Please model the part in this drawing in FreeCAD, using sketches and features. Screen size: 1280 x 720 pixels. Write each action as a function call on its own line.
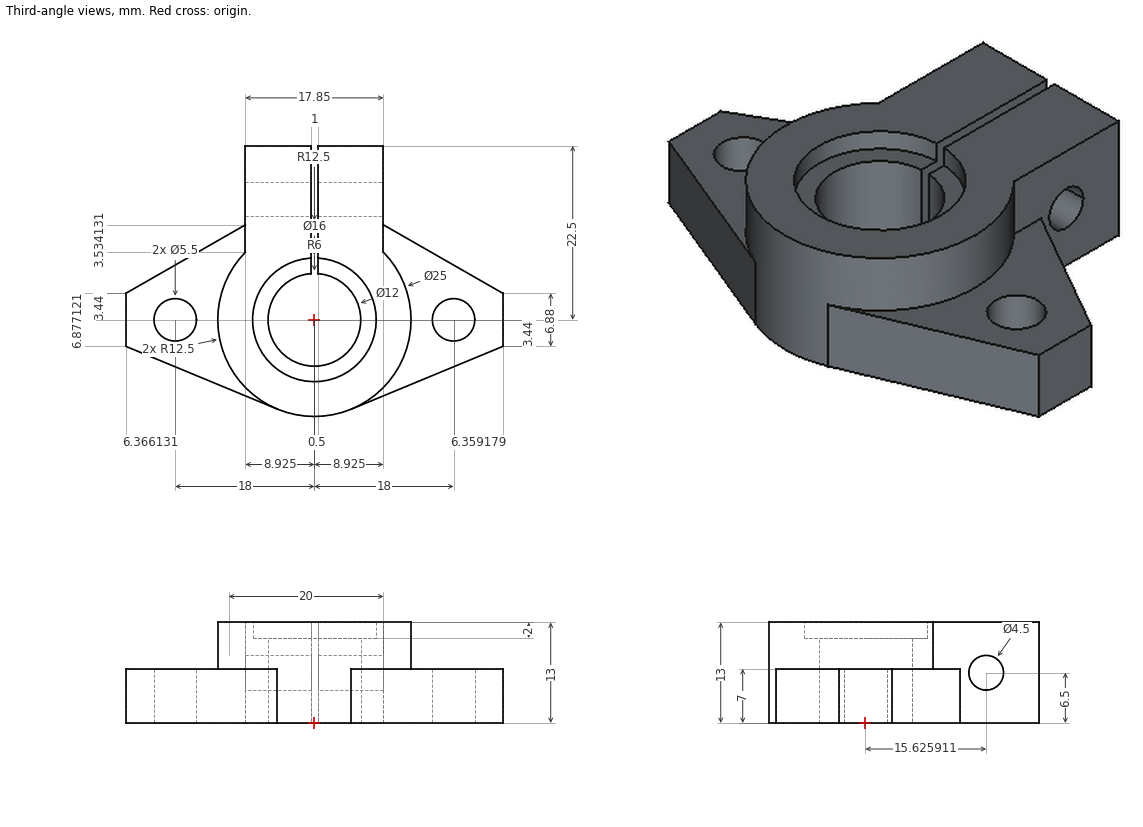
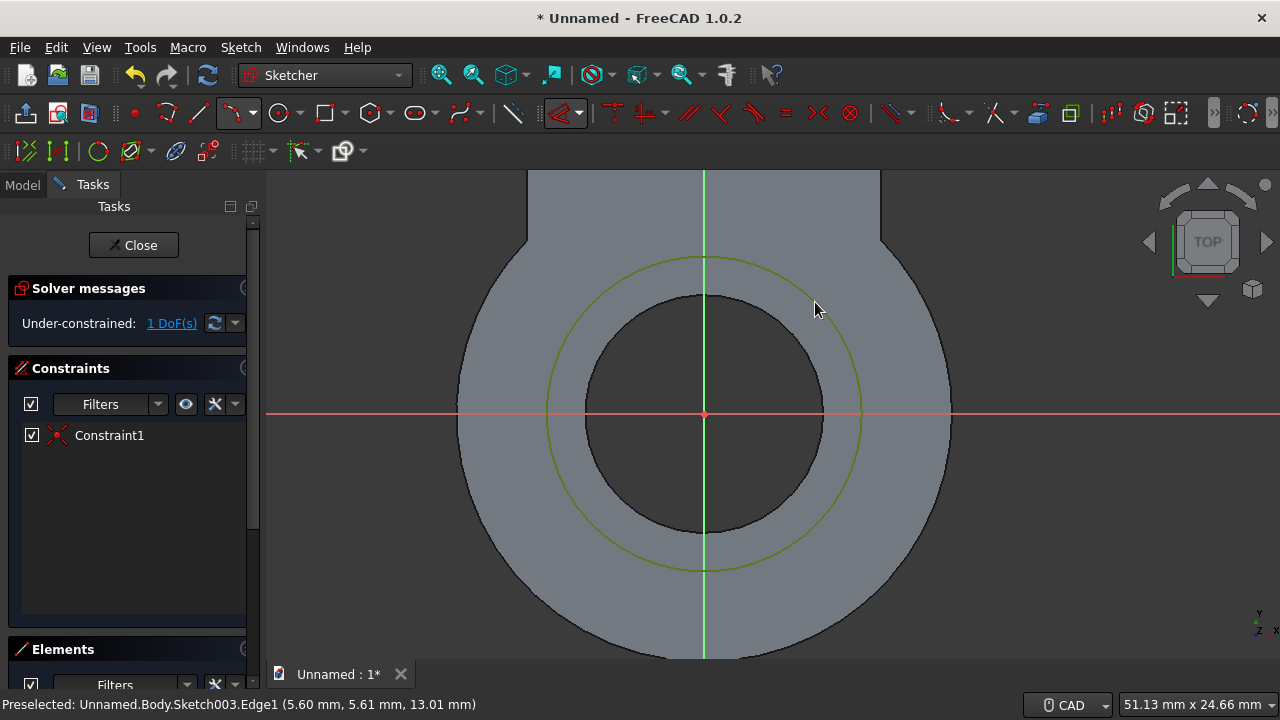
click(582, 114)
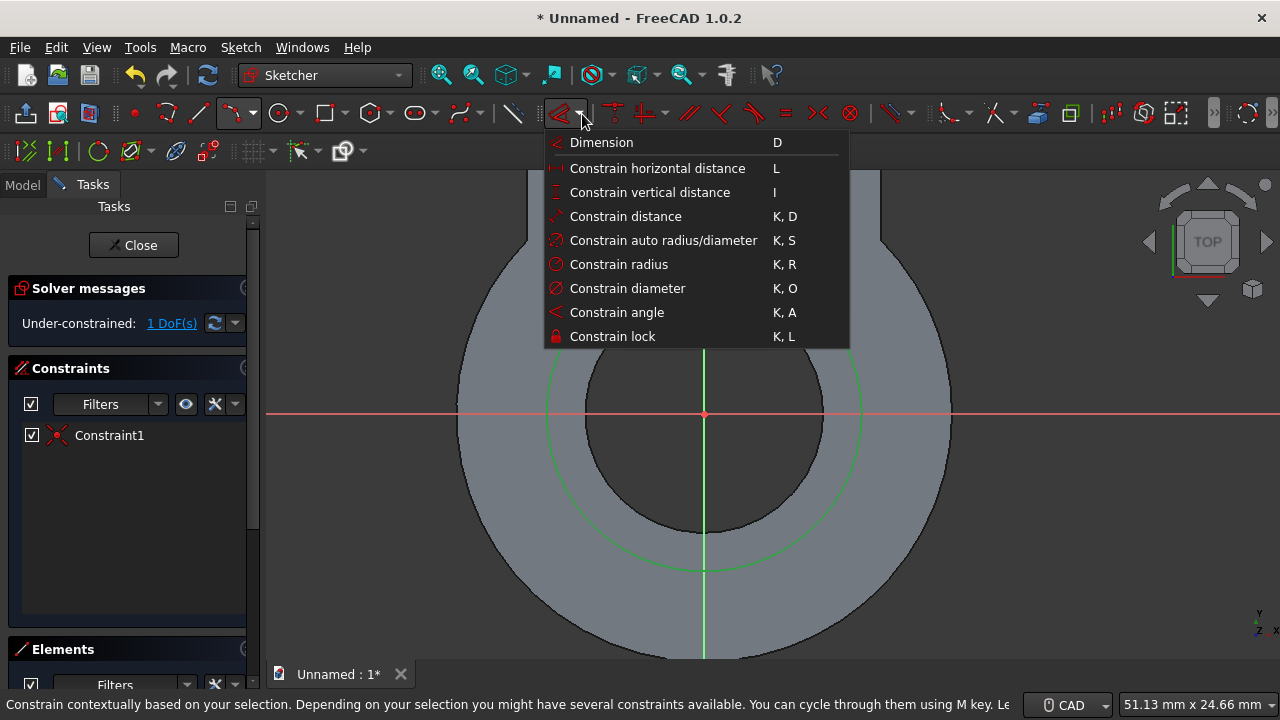
click(697, 288)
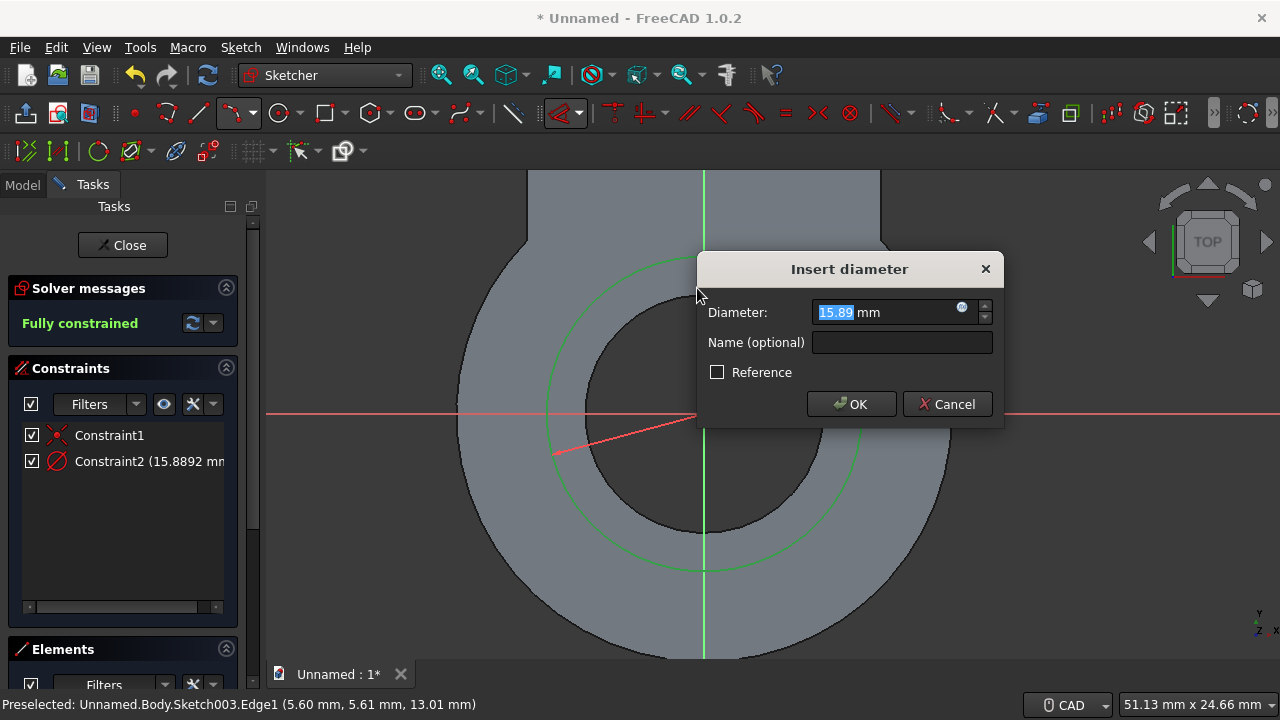
text(16)
key(Return)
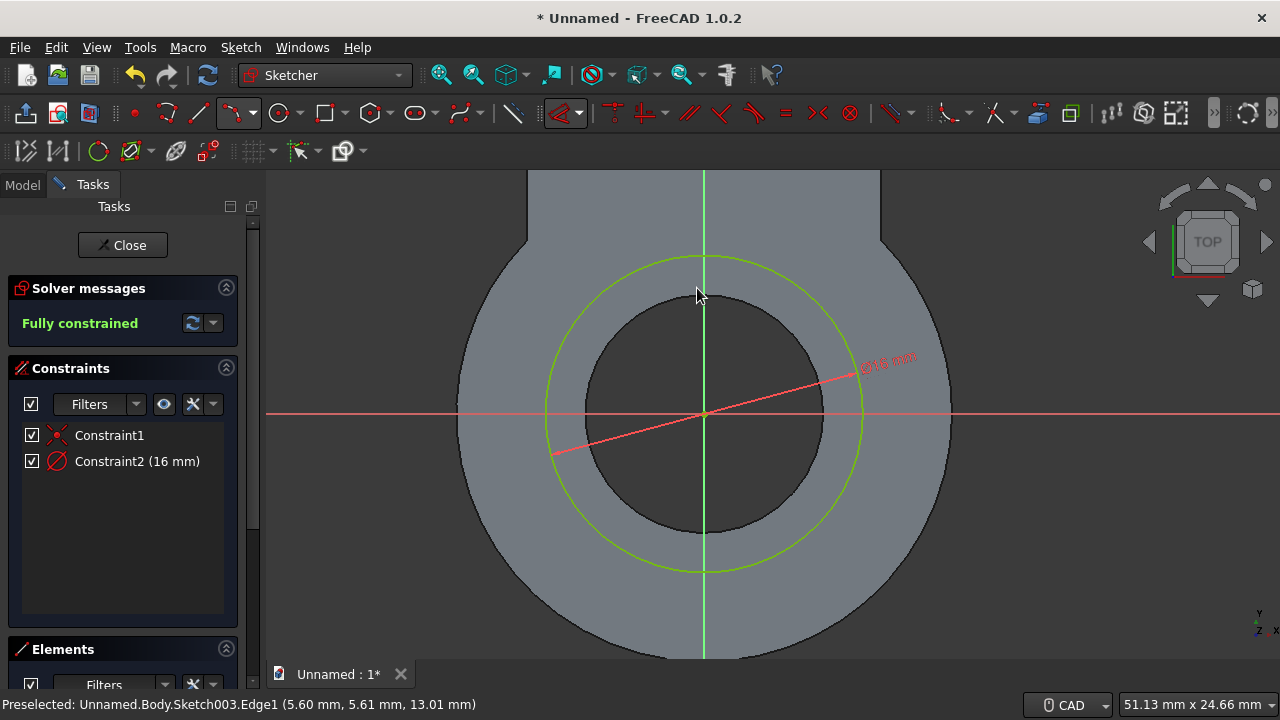
click(123, 245)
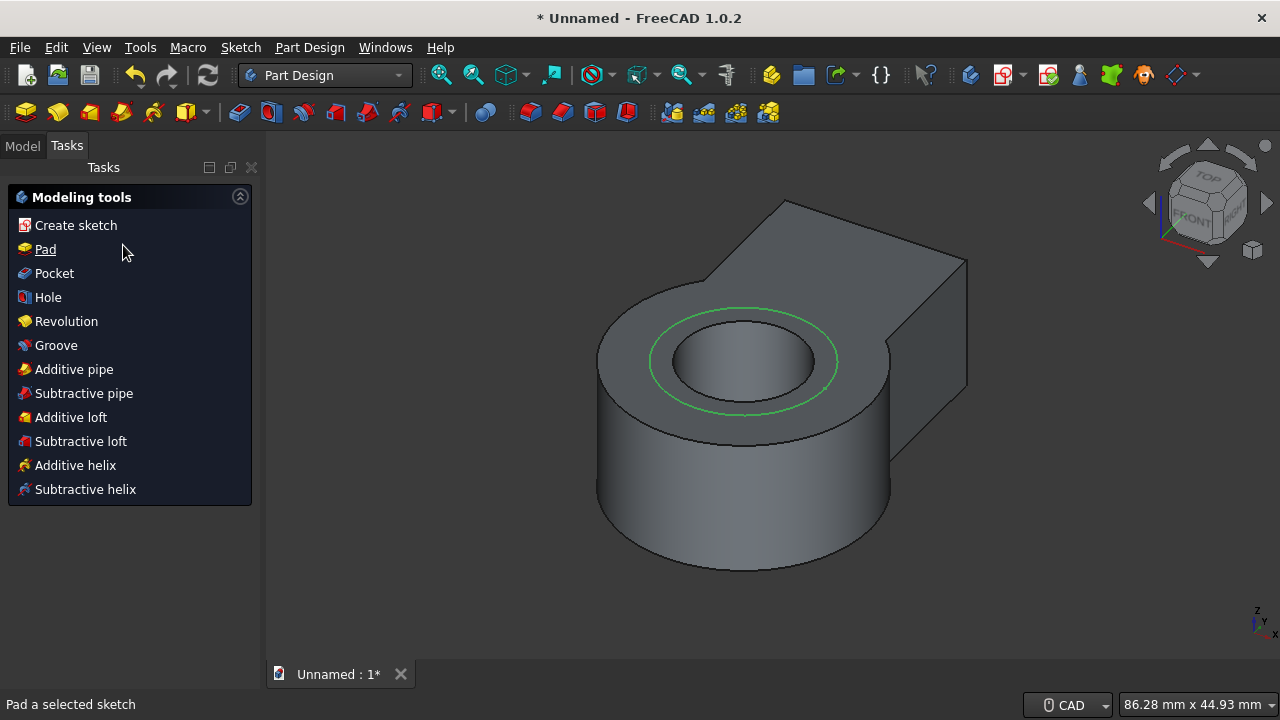
click(240, 112)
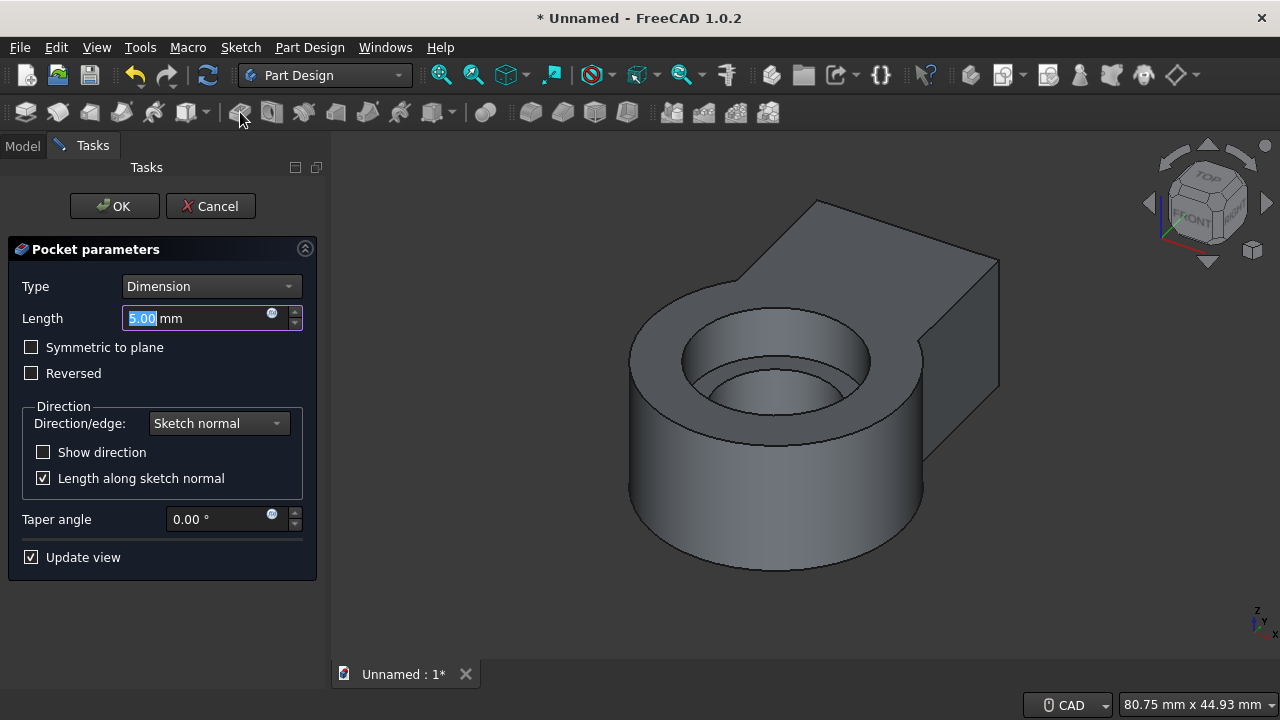
text(2)
key(Tab)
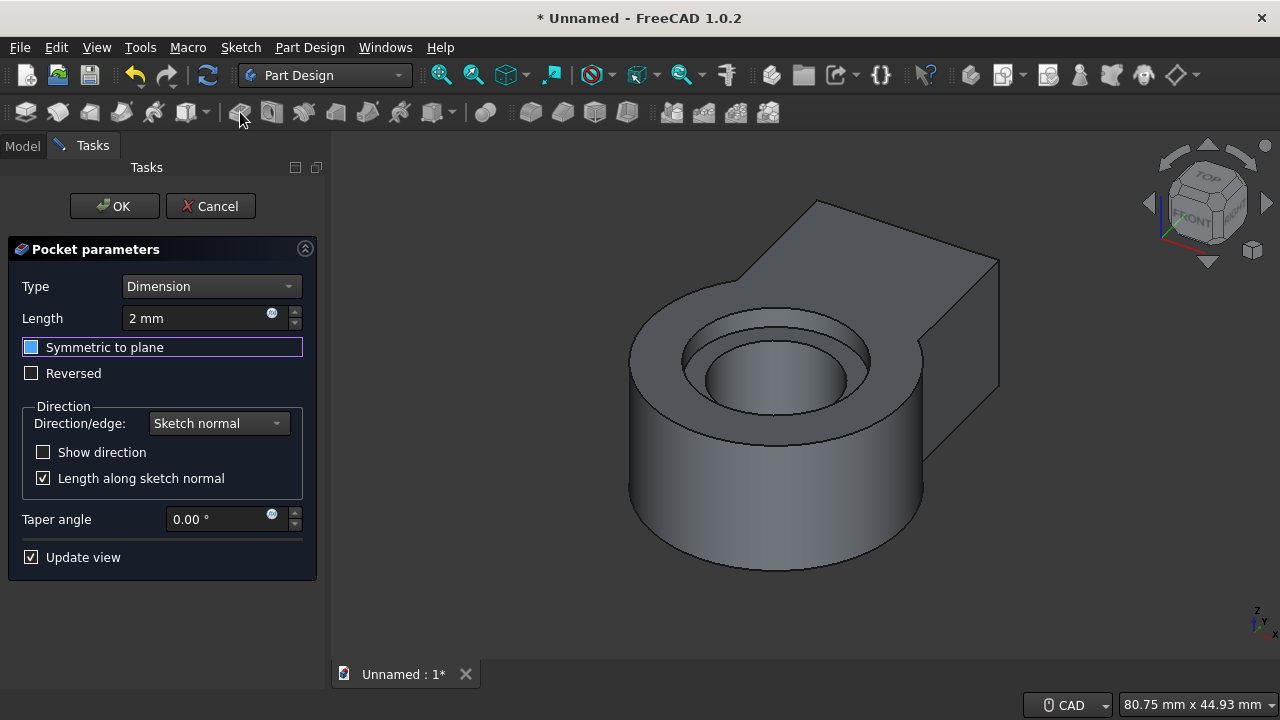
click(115, 206)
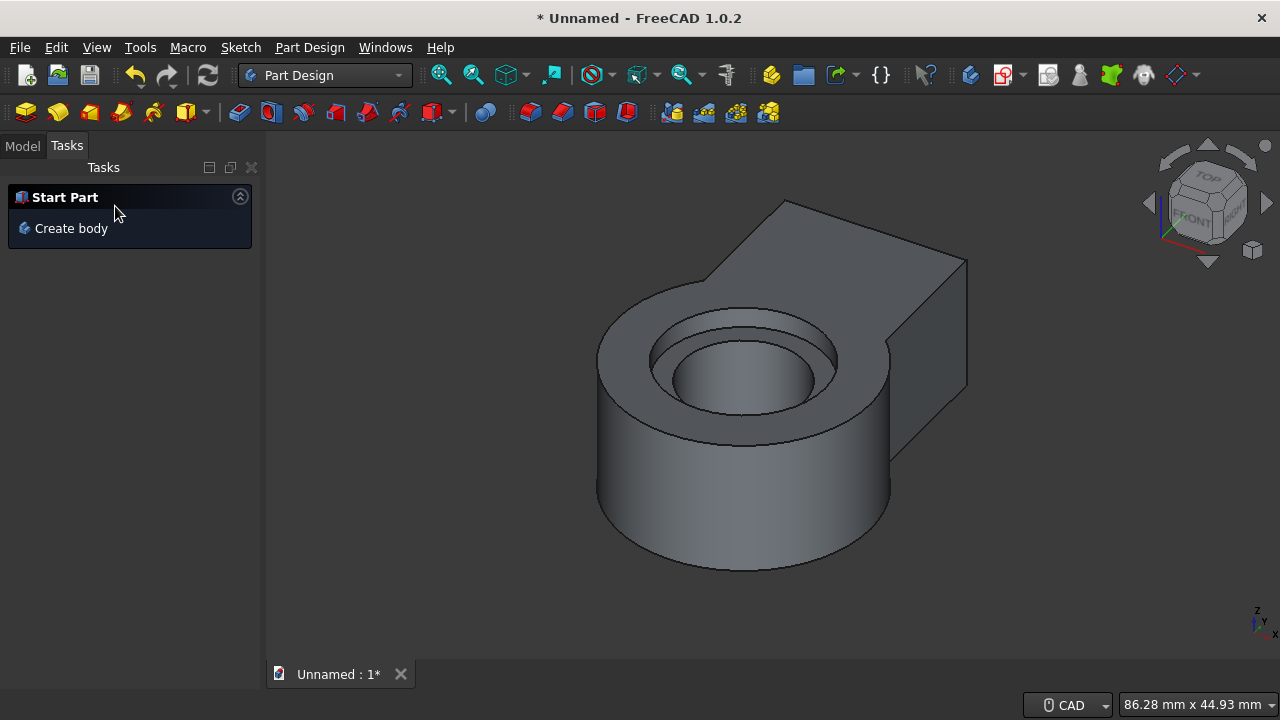
key(5)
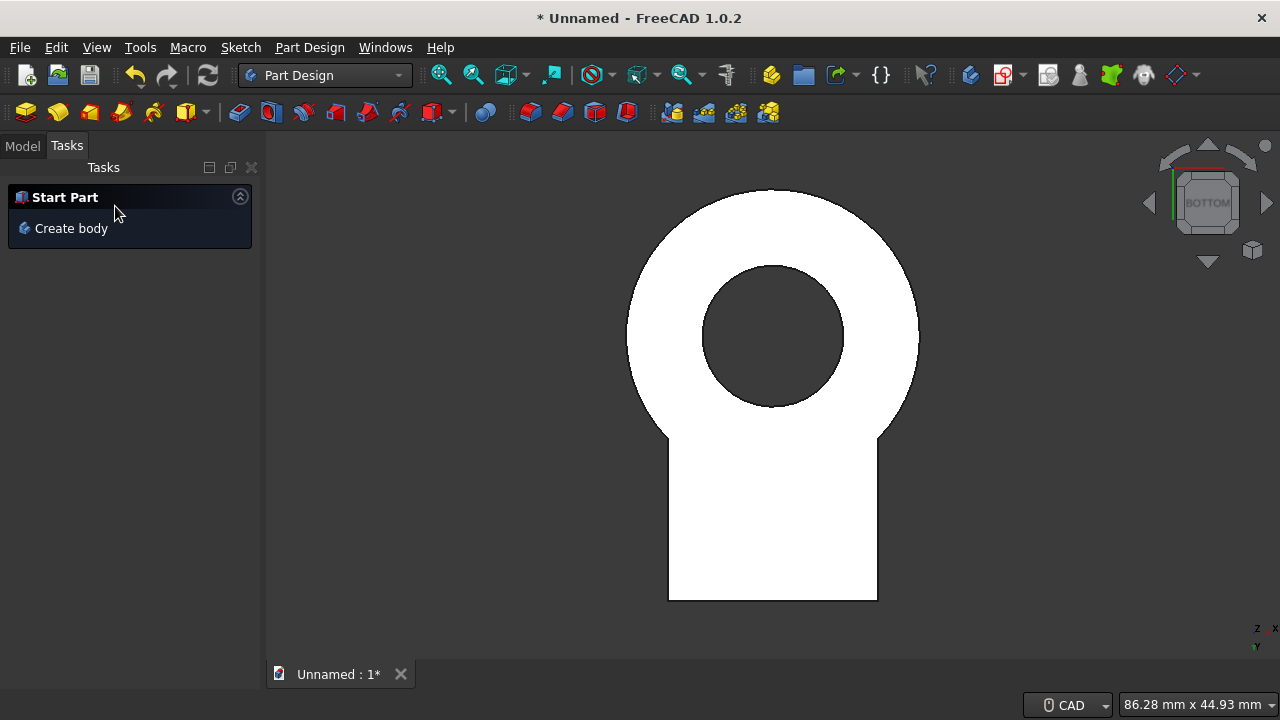
click(773, 512)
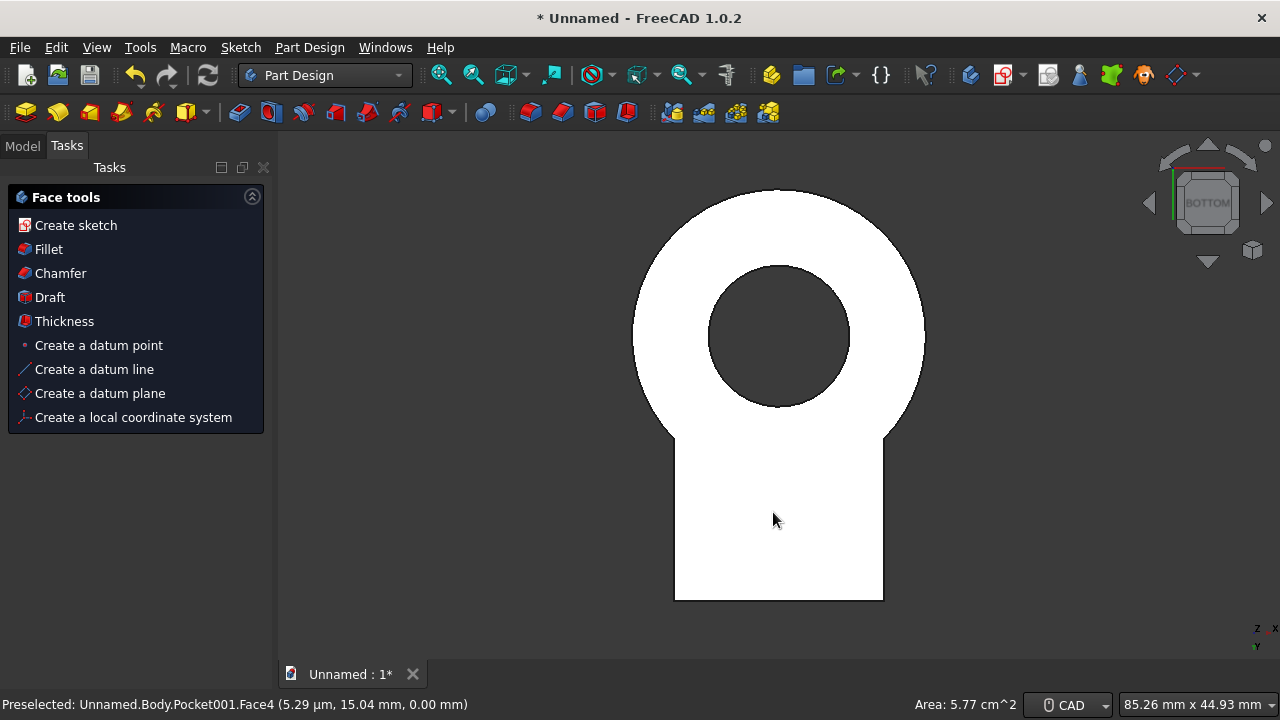
click(1004, 76)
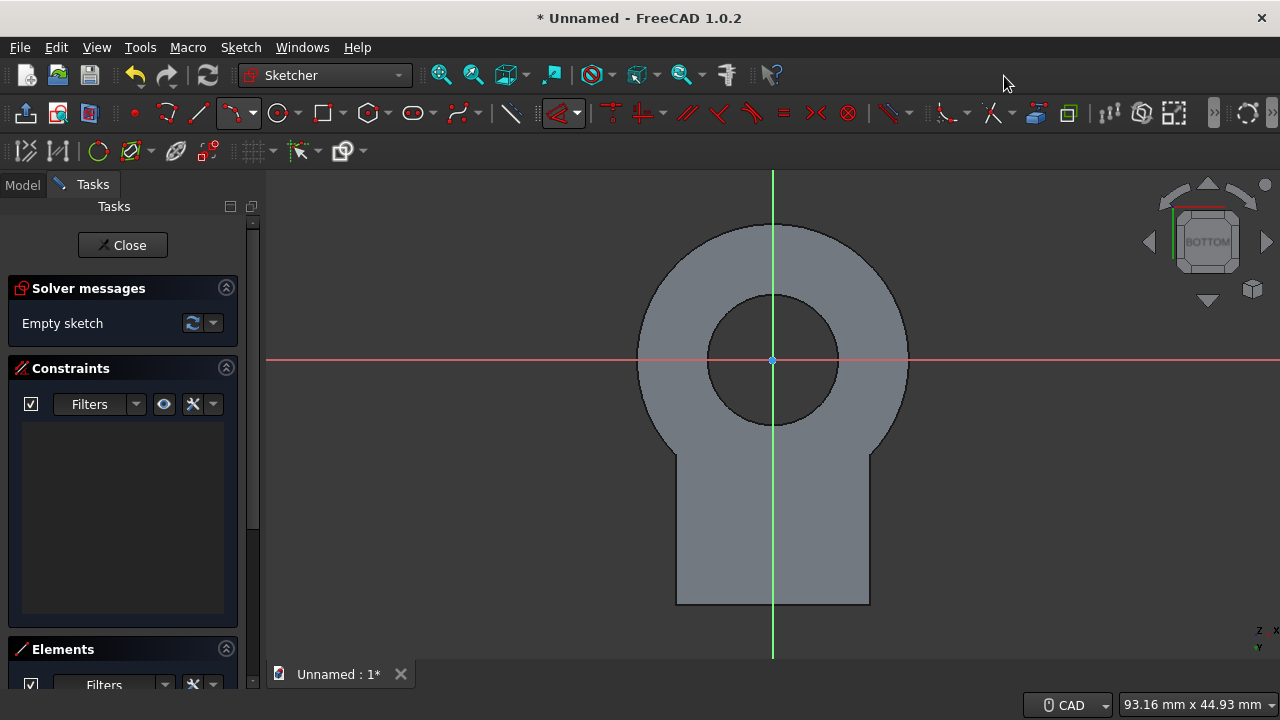
click(168, 114)